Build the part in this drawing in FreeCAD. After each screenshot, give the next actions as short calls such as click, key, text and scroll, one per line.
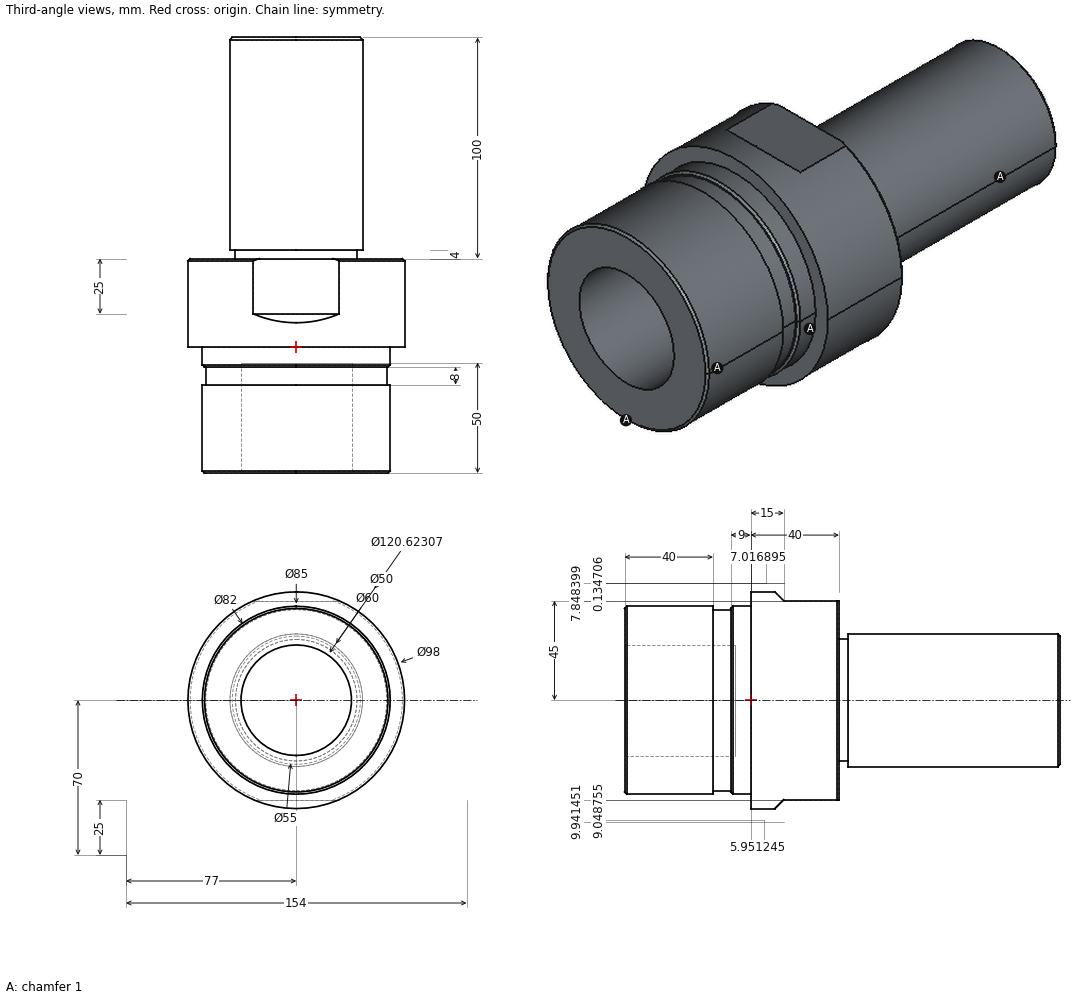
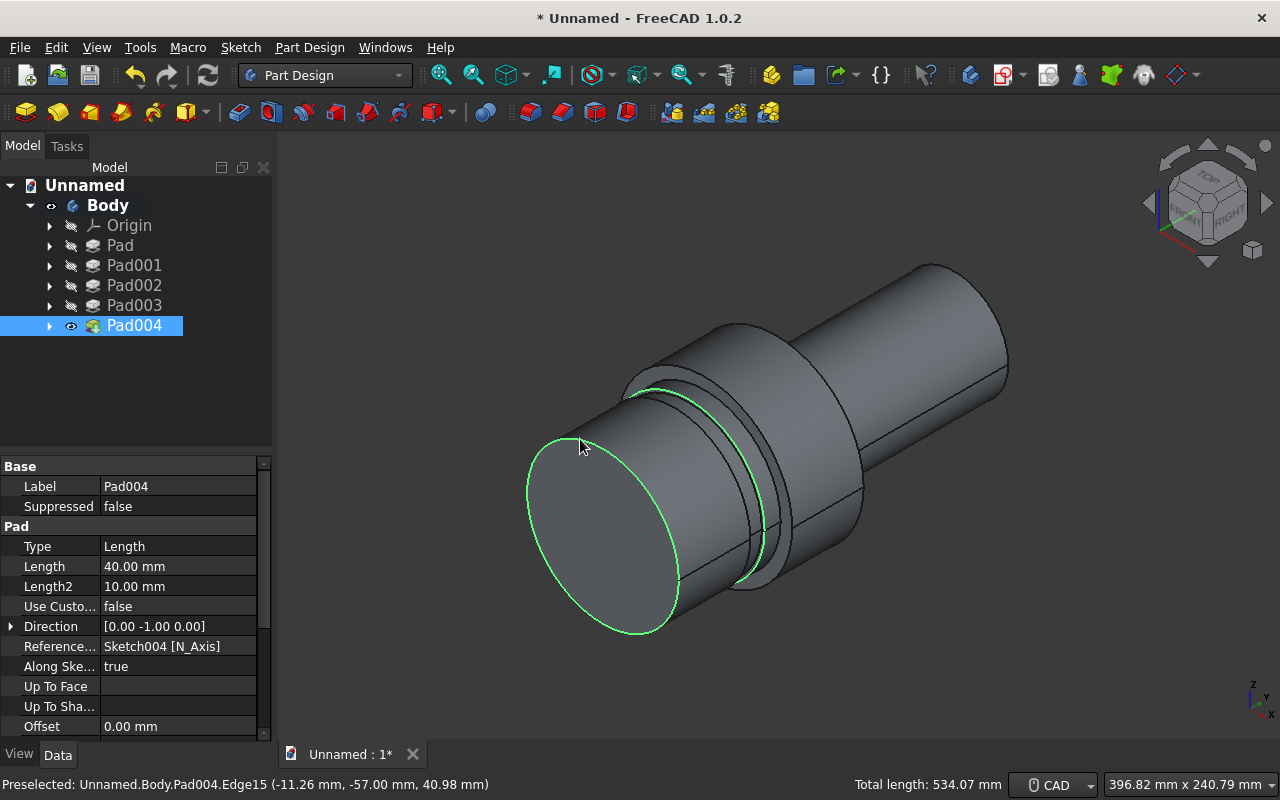
key(2)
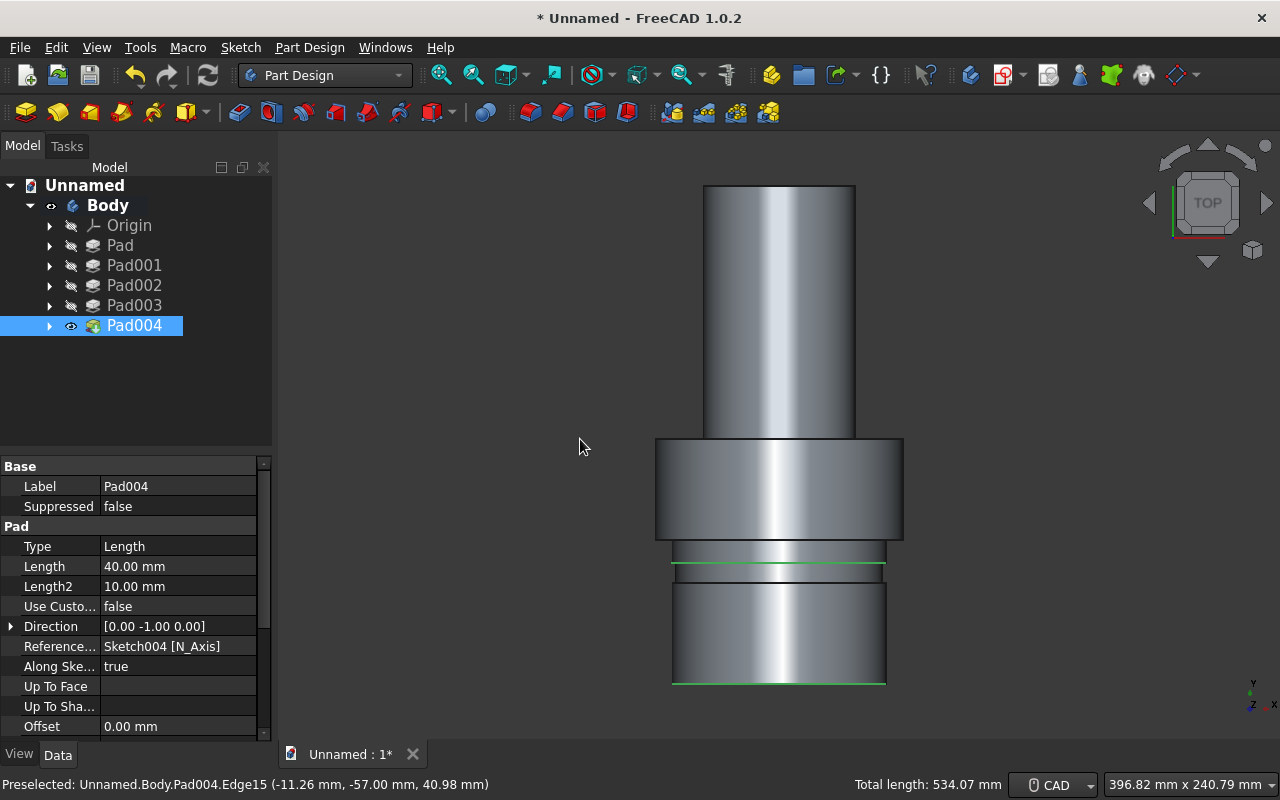
click(679, 438, ctrl)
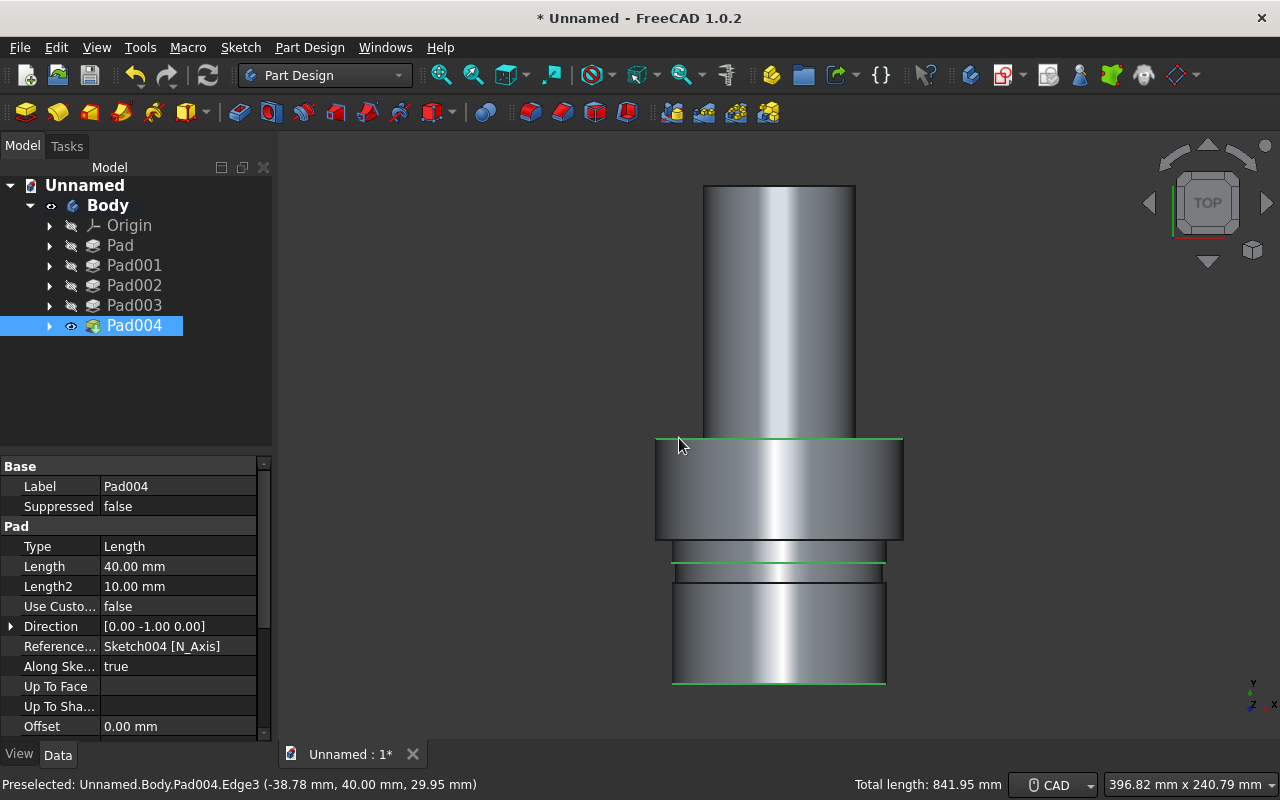
click(718, 185, ctrl)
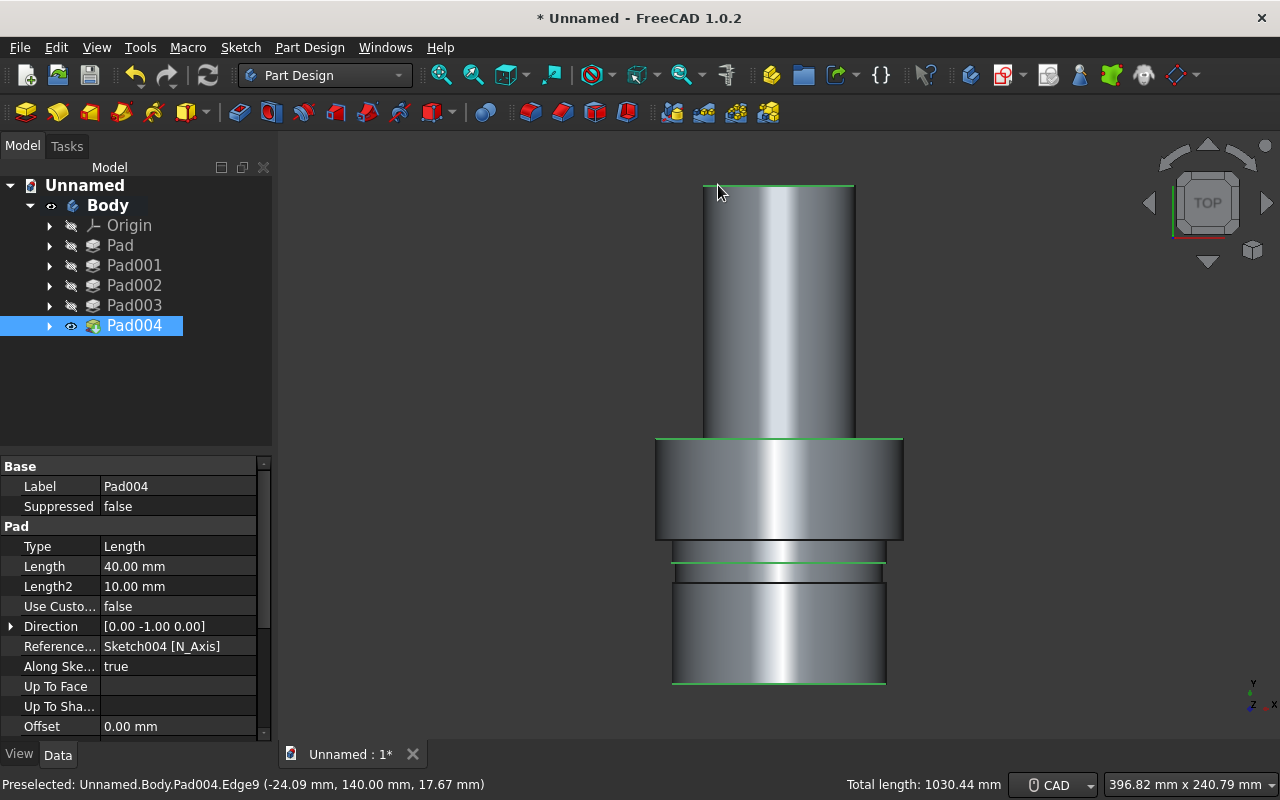
click(564, 112)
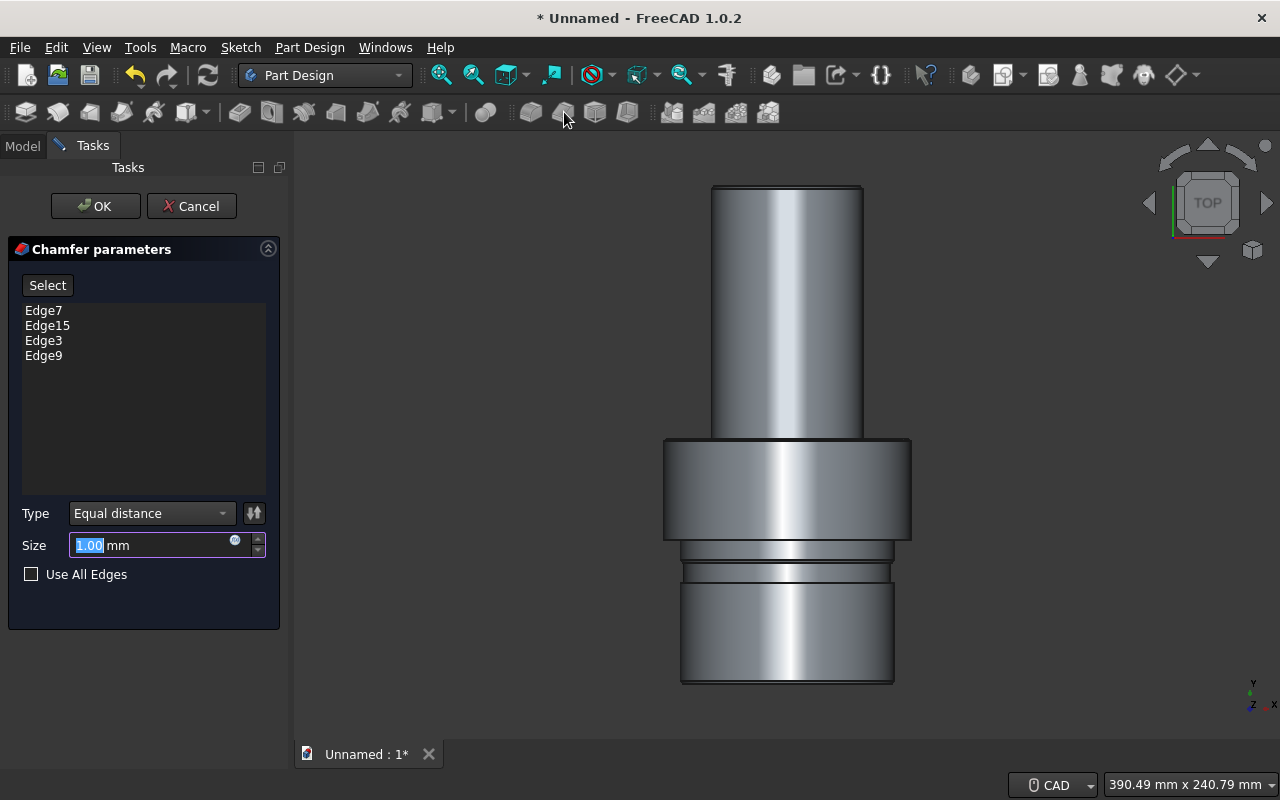
text(1)
key(Tab)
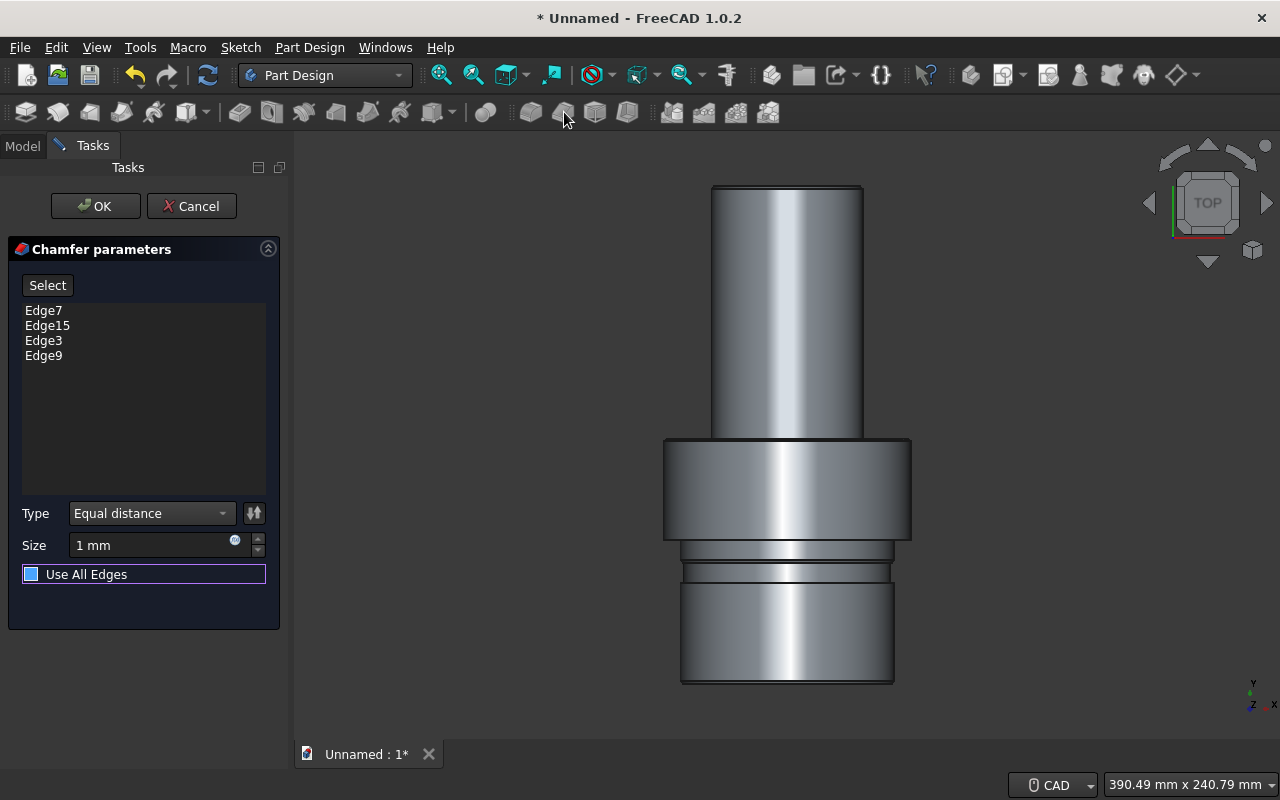
click(96, 206)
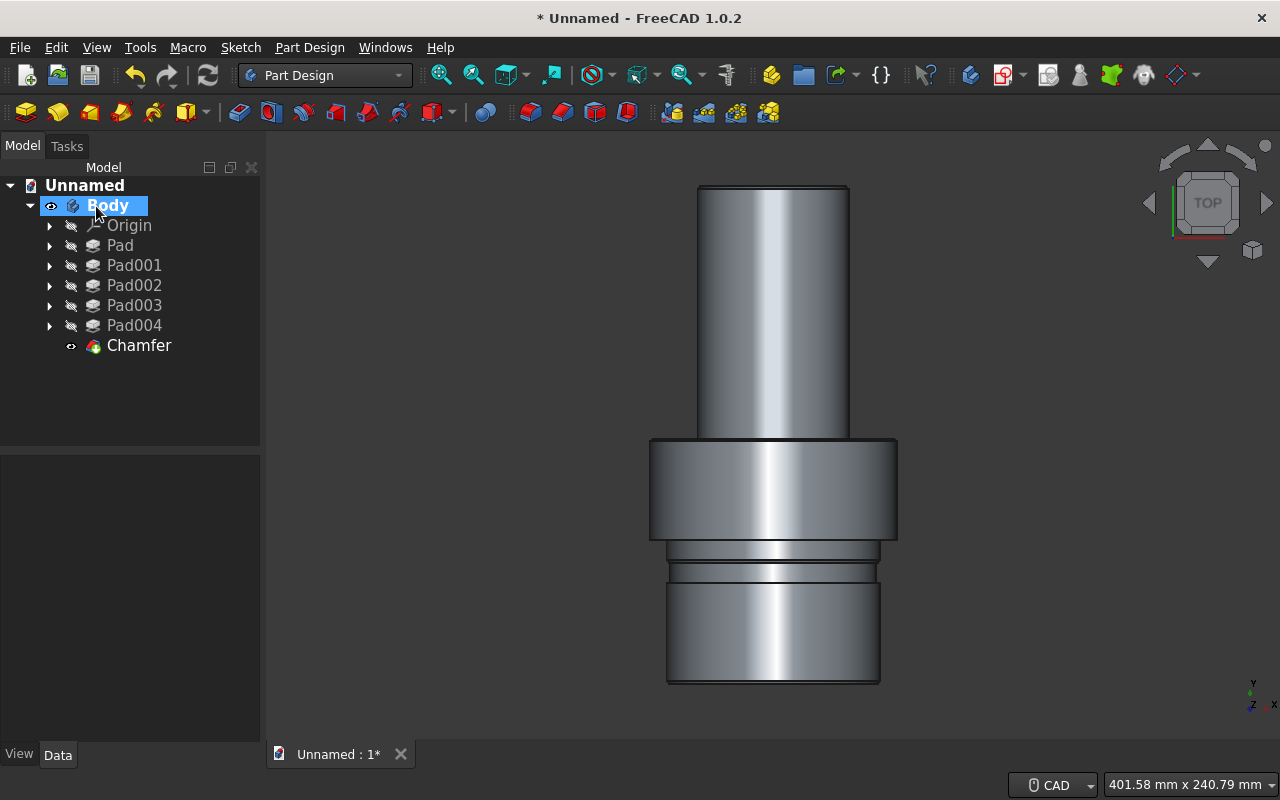
key(4)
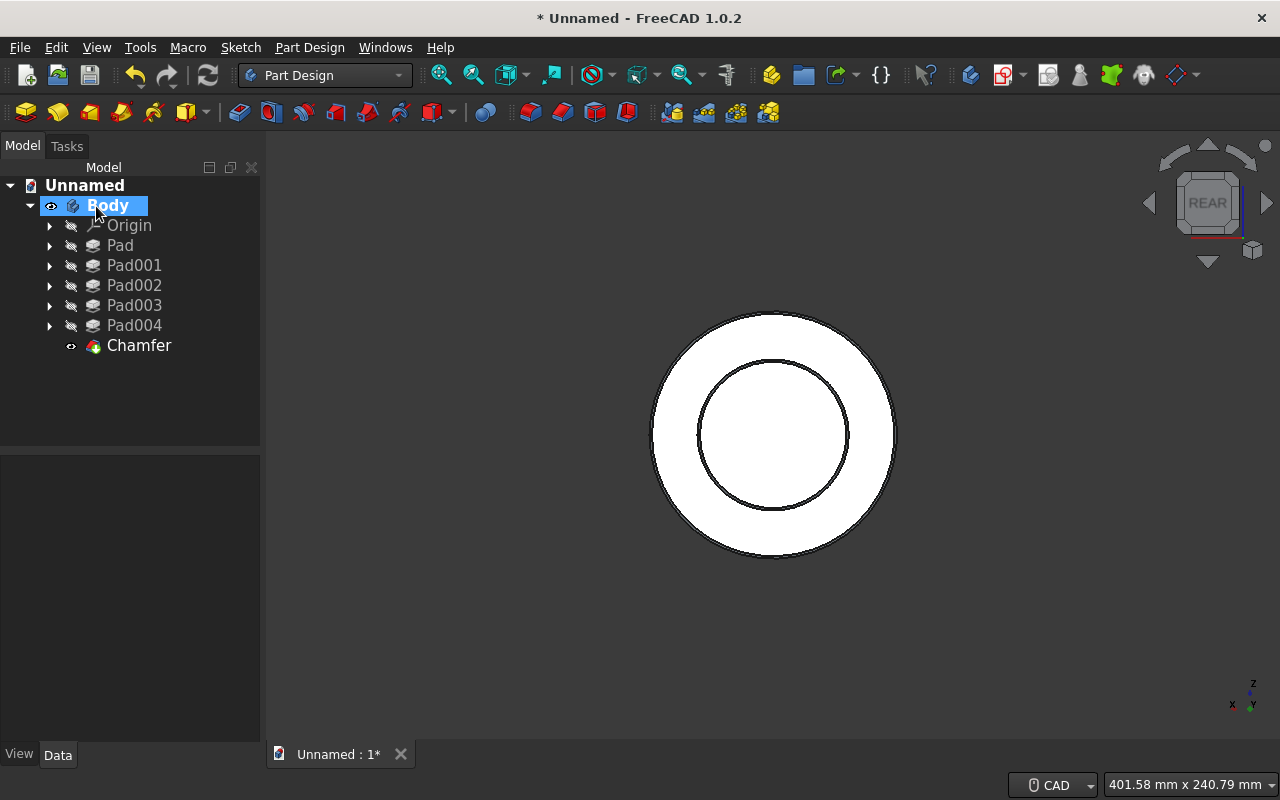
click(442, 76)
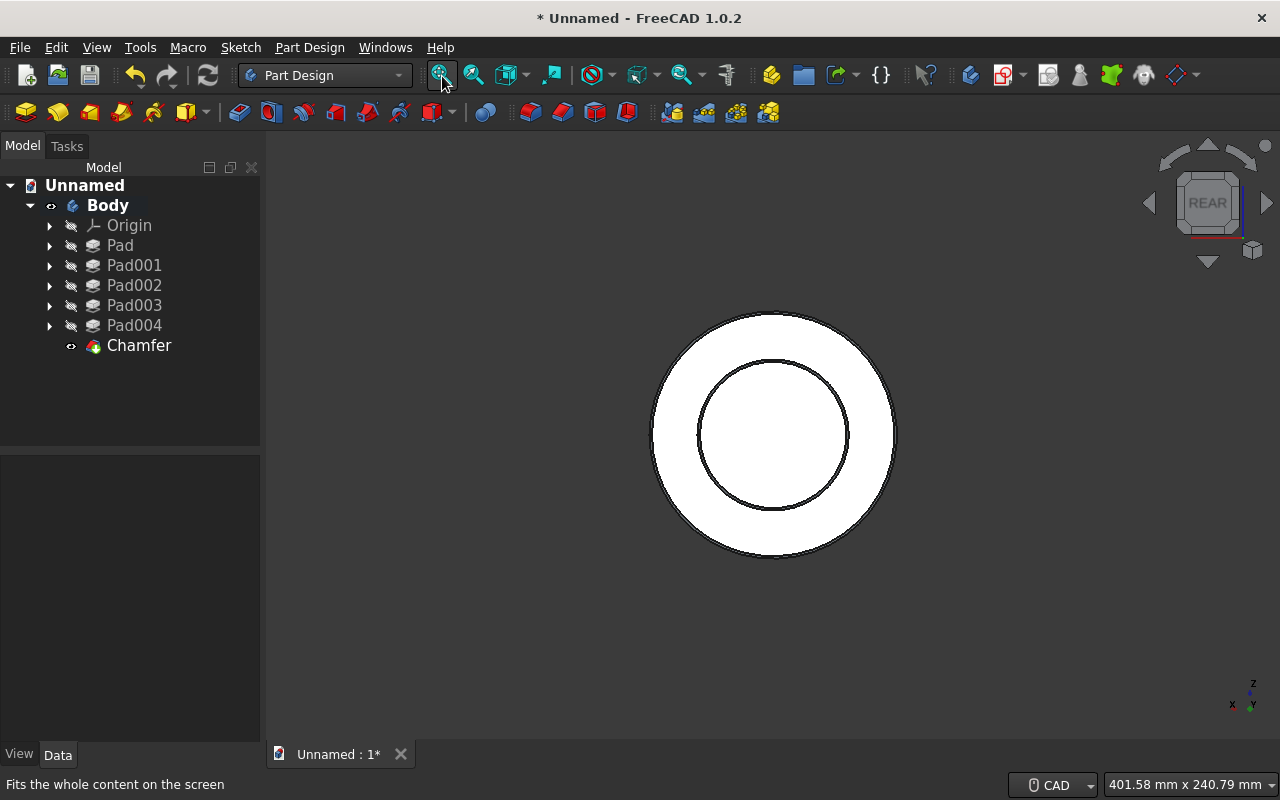
click(842, 503)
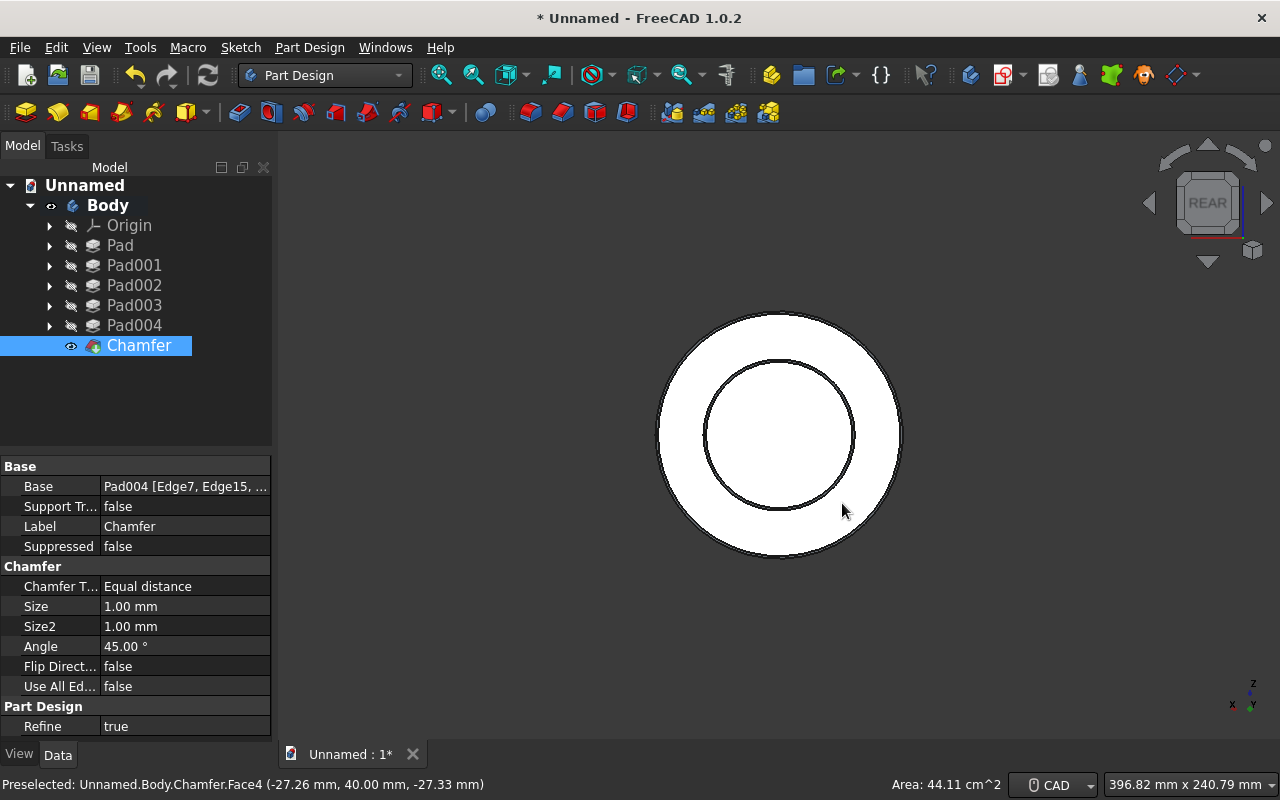
click(1004, 76)